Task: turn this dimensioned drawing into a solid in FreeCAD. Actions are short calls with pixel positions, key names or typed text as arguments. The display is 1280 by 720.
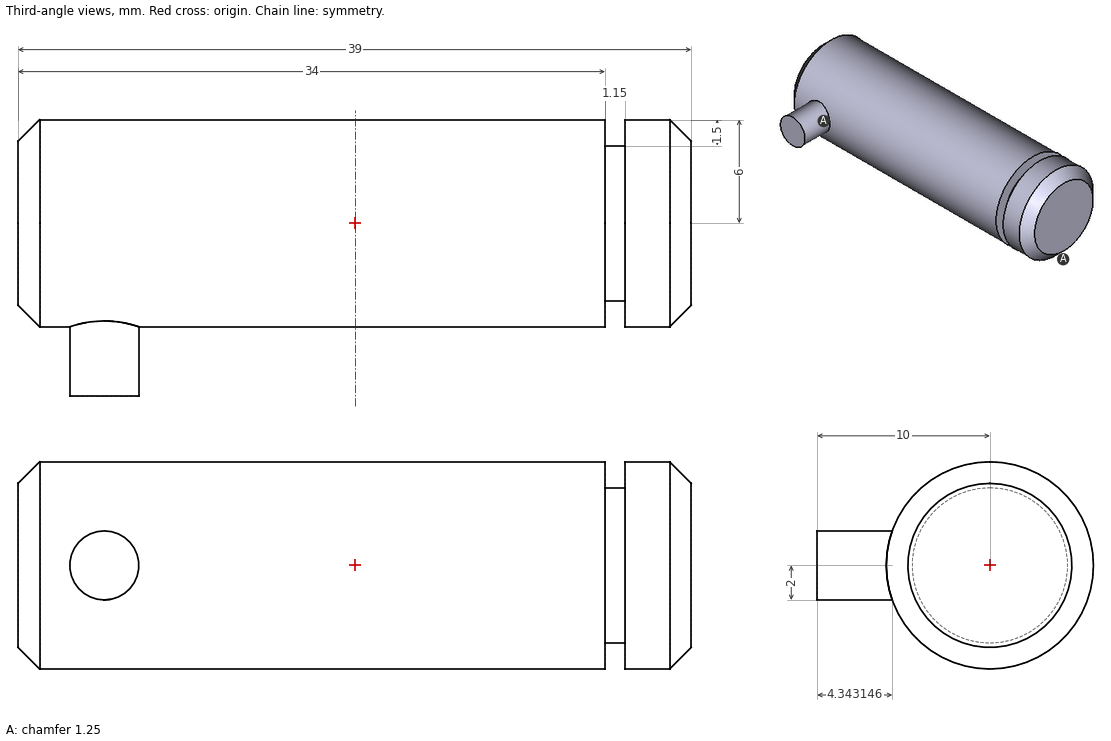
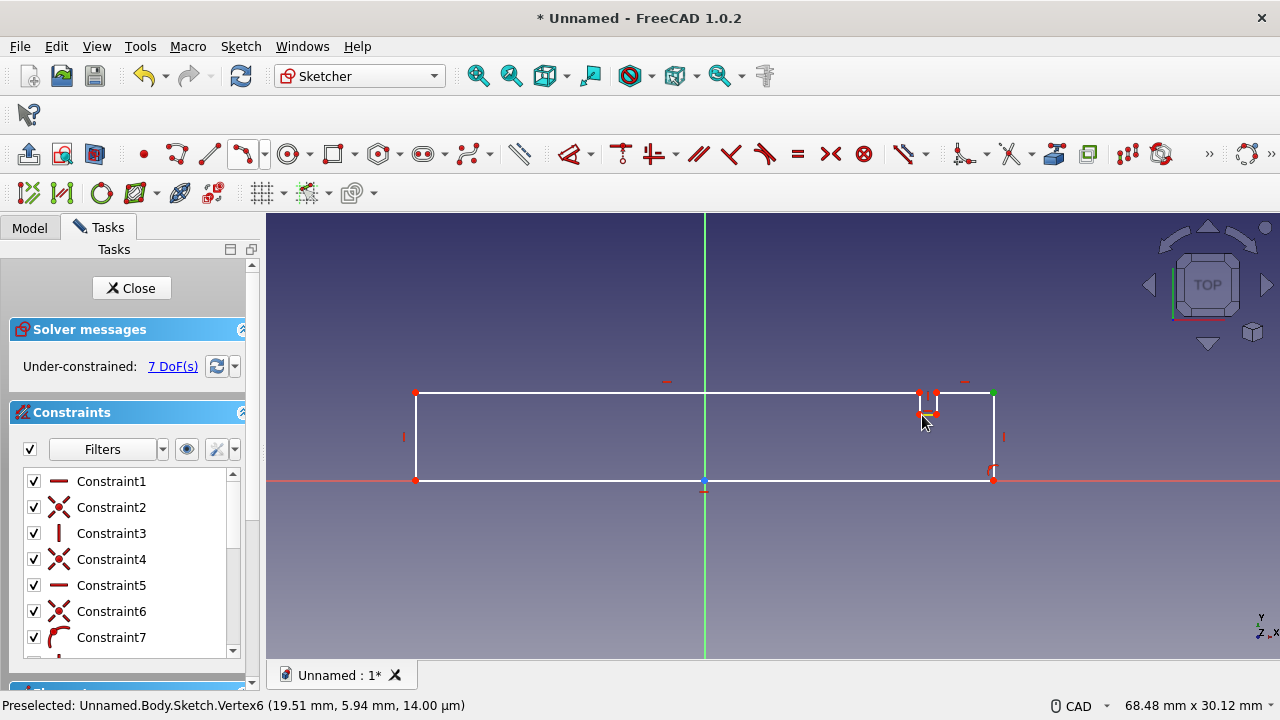
click(416, 393)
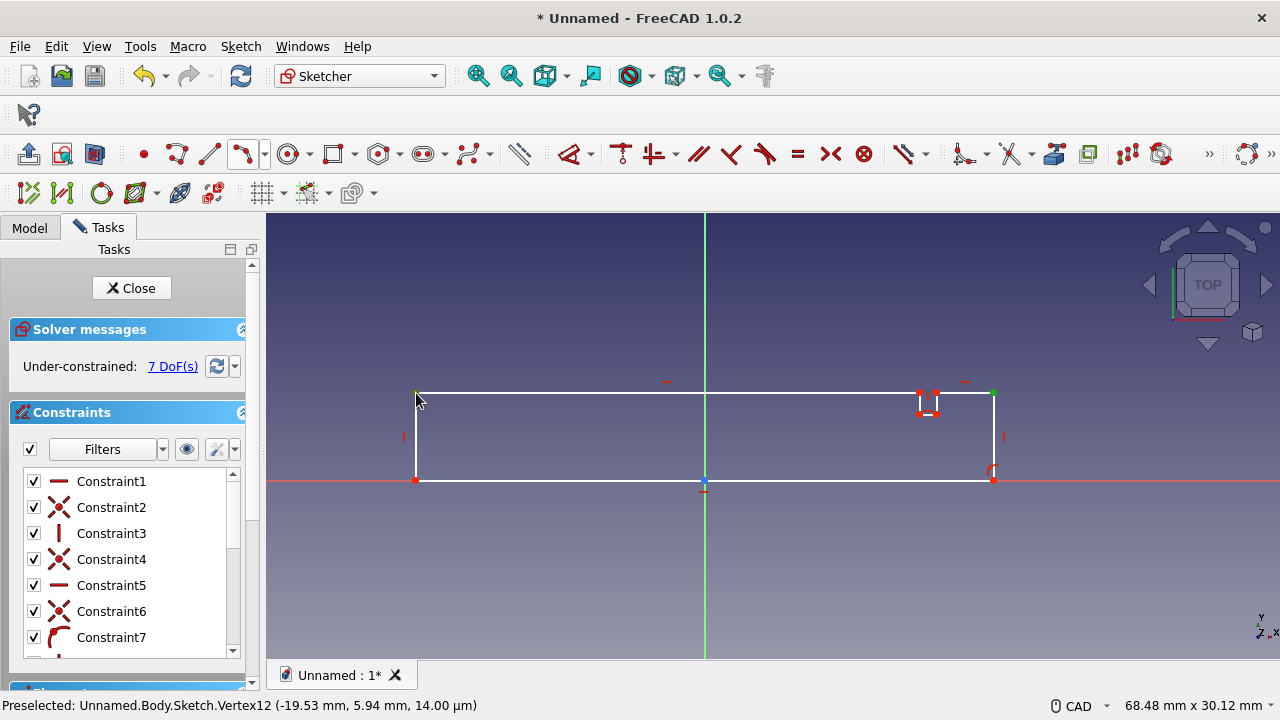
click(705, 603)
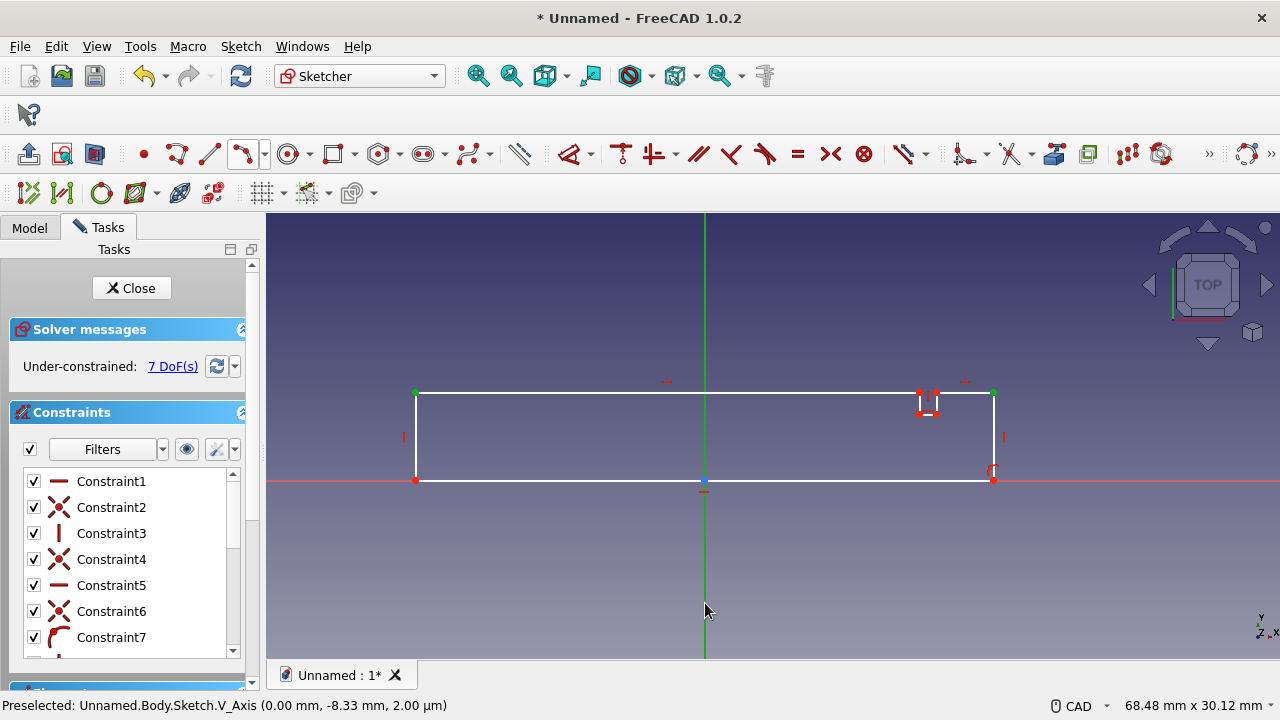
click(831, 154)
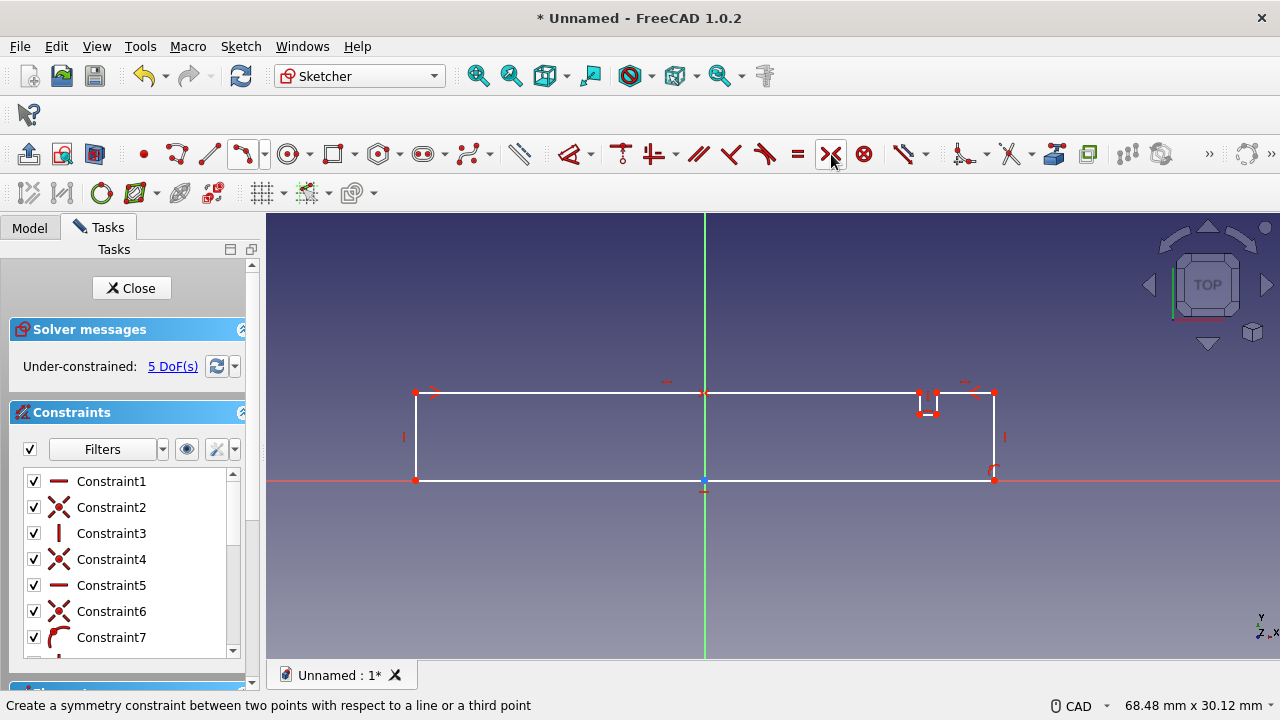
click(994, 419)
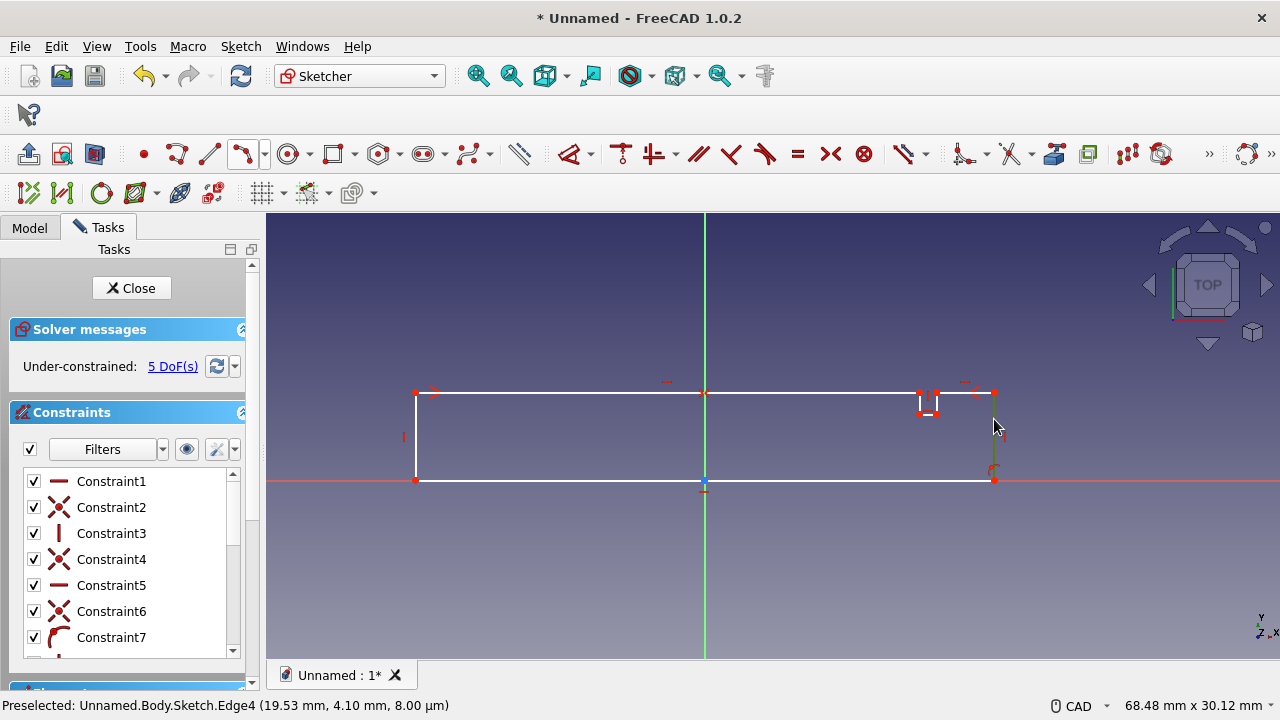
key(i)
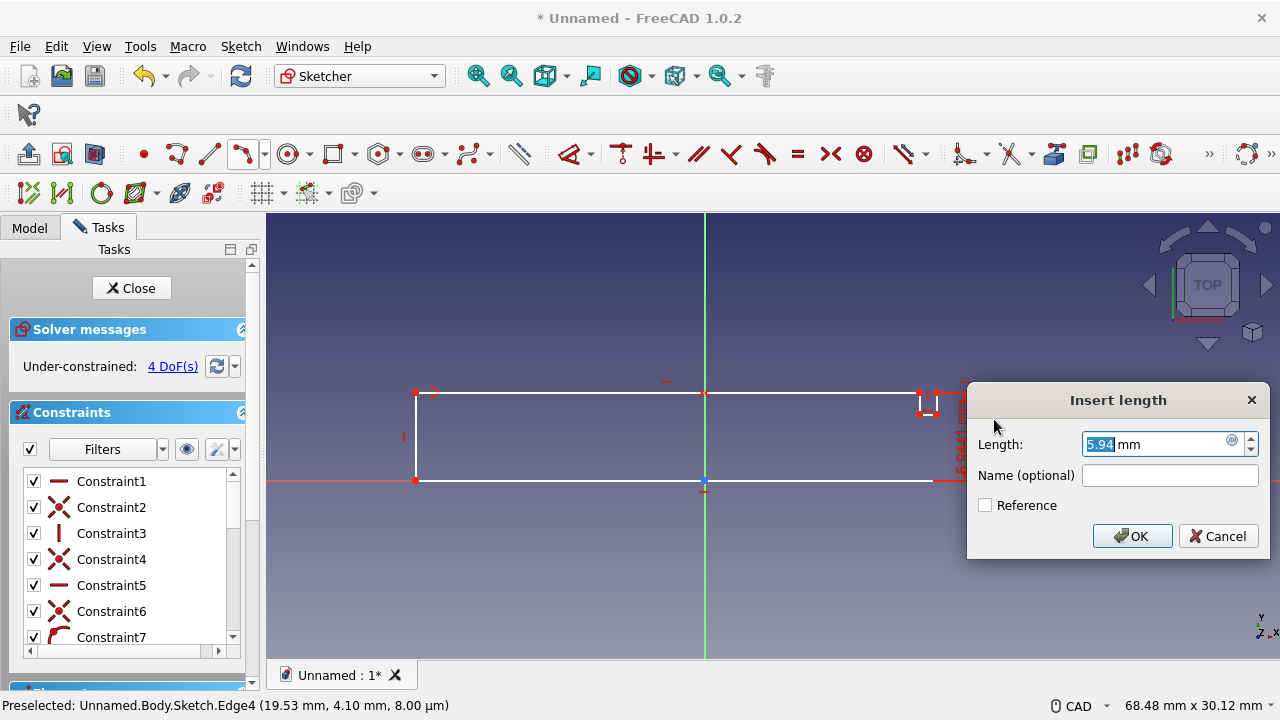
text(6)
key(Return)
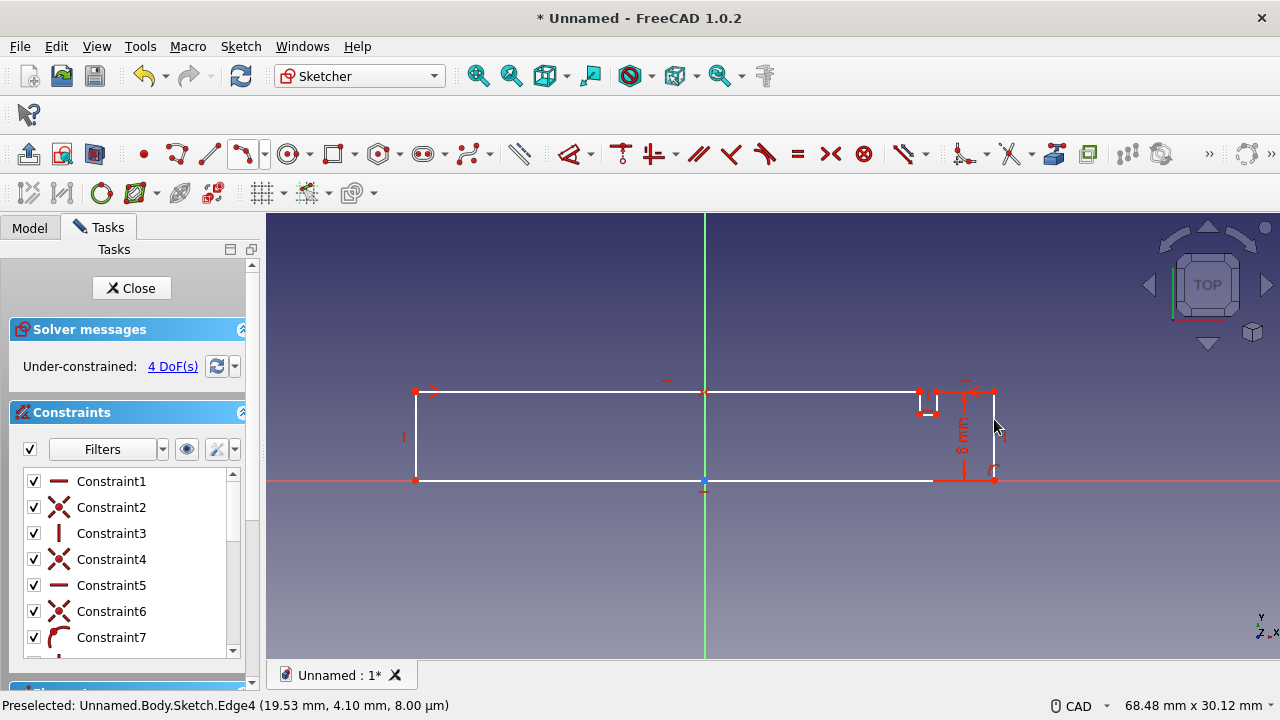
click(821, 481)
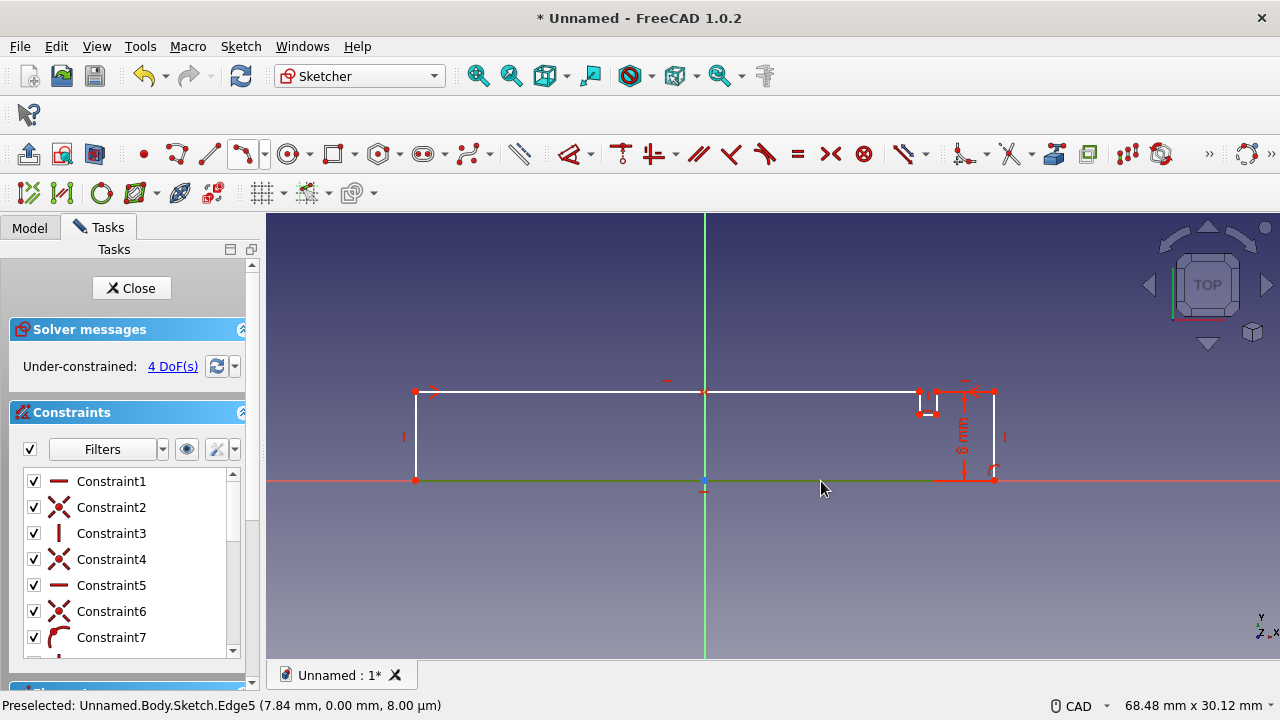
key(l)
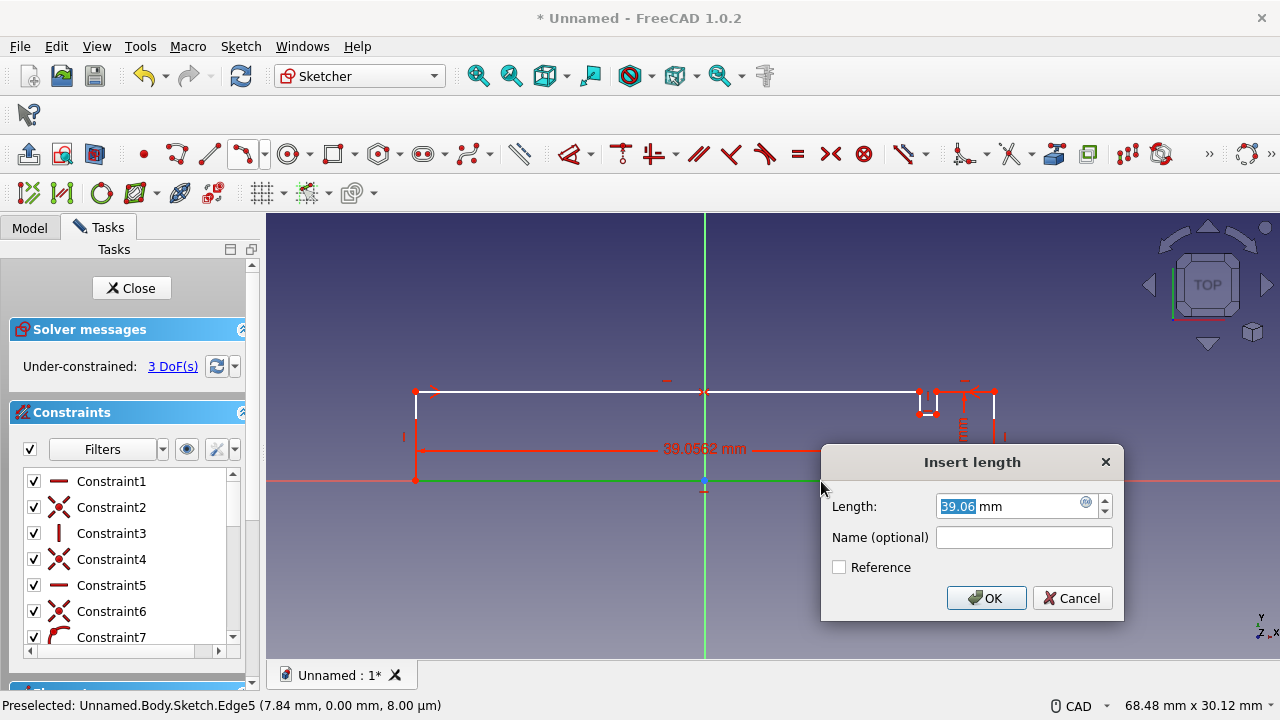
text(39)
key(Return)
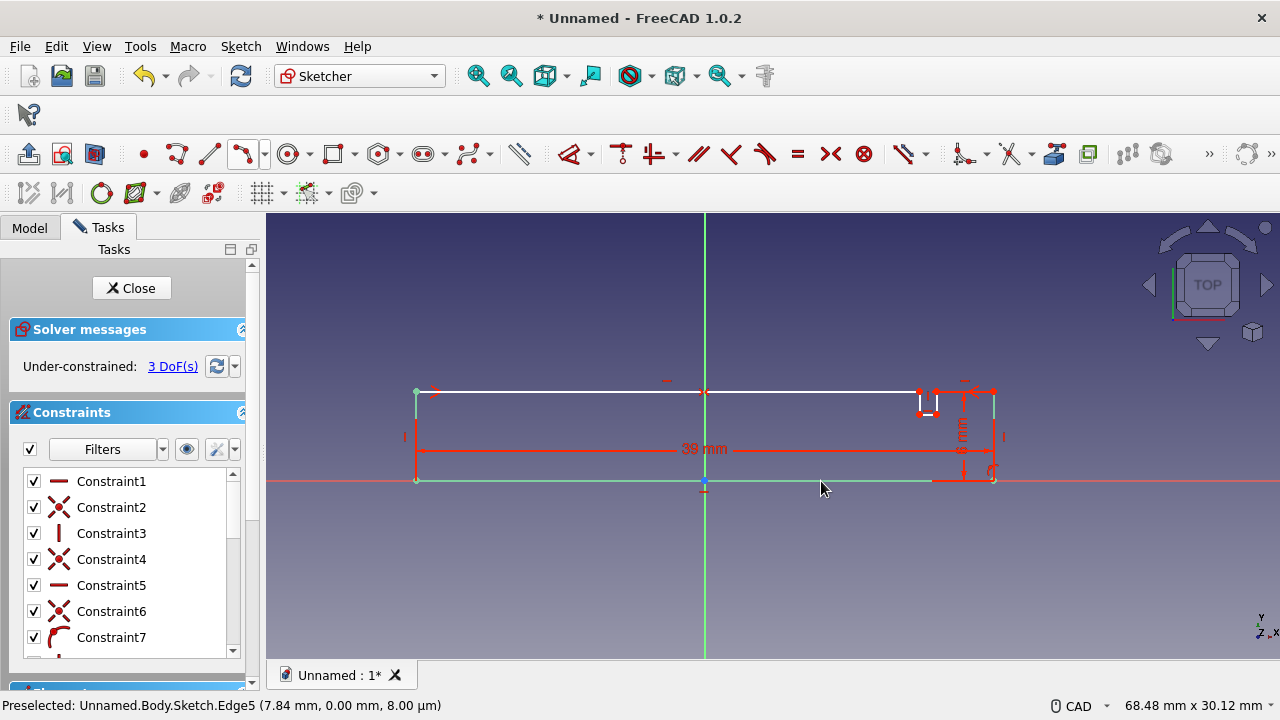
click(567, 392)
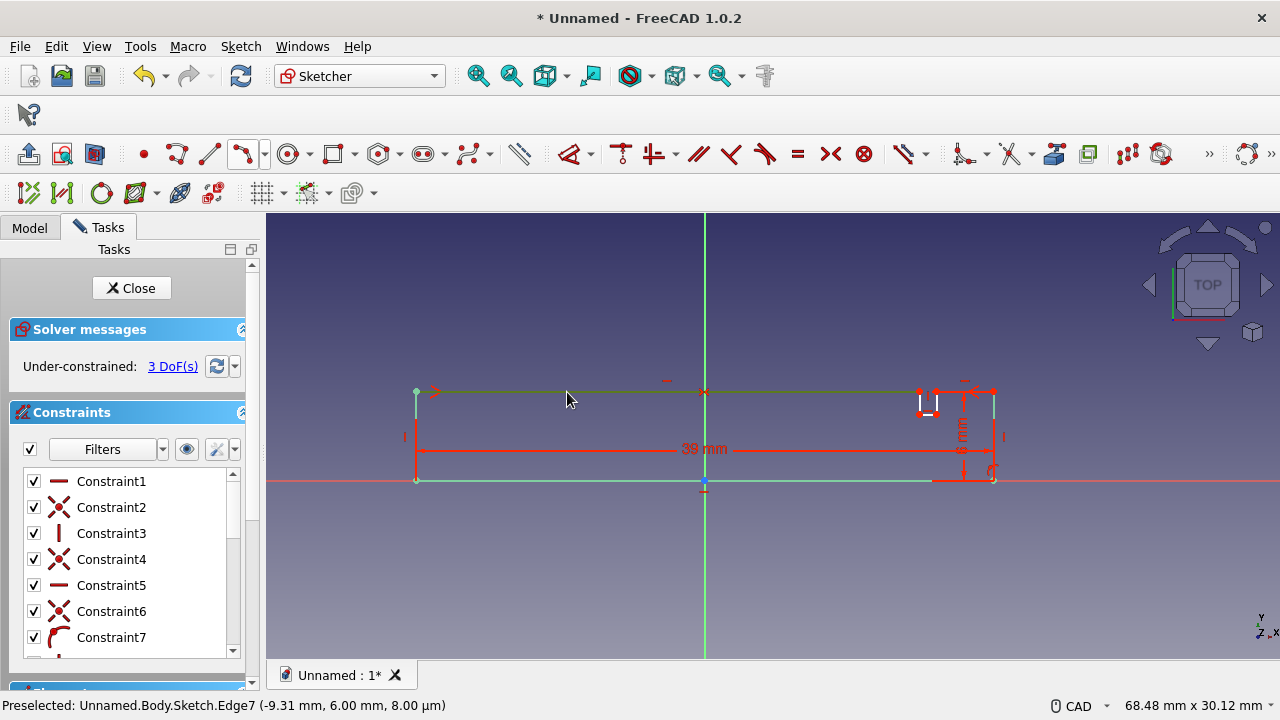
key(l)